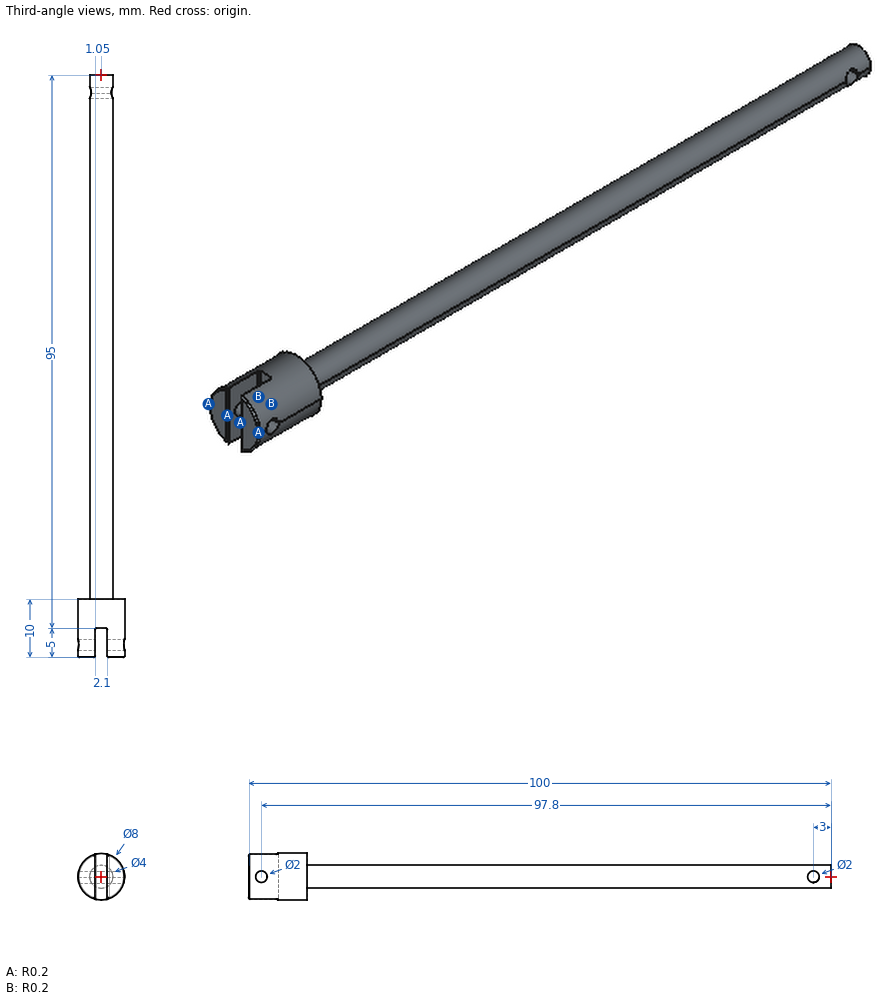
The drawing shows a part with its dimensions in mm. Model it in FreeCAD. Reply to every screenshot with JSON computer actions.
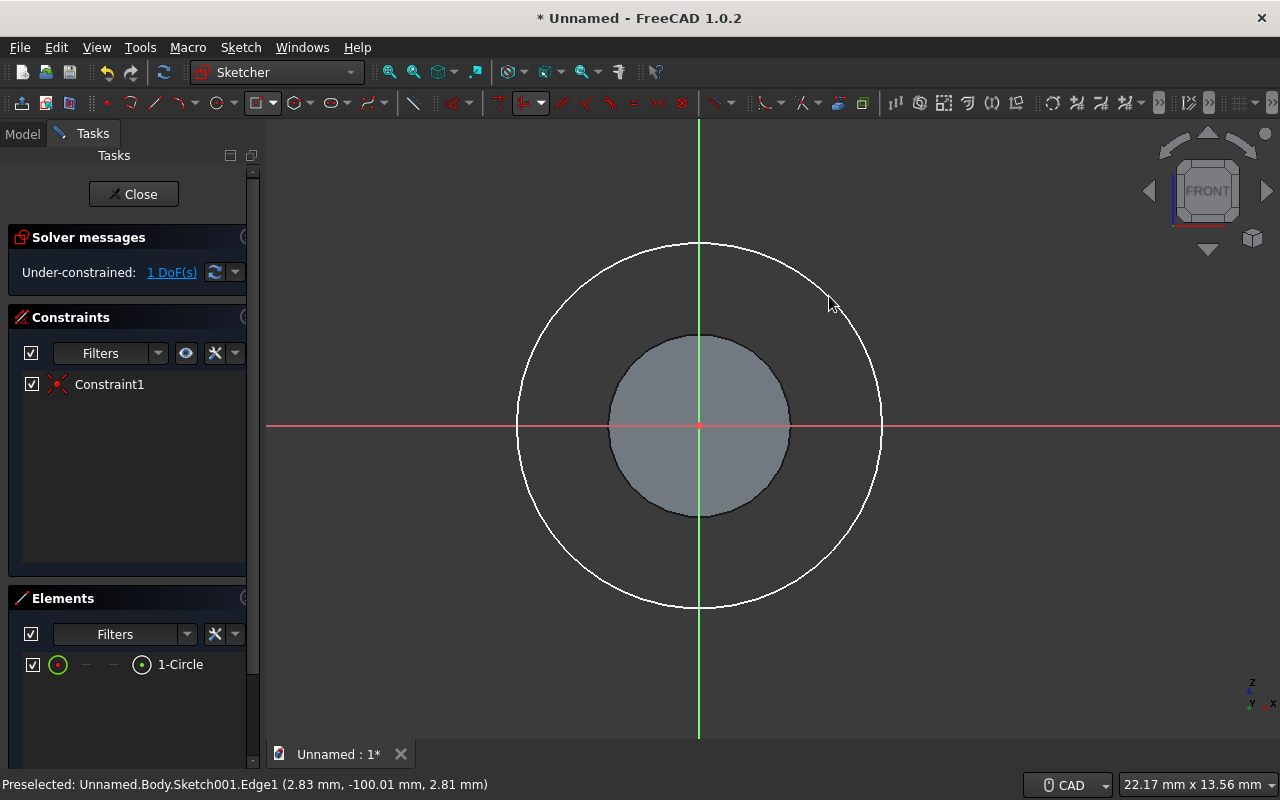
{"action": "key", "text": "d"}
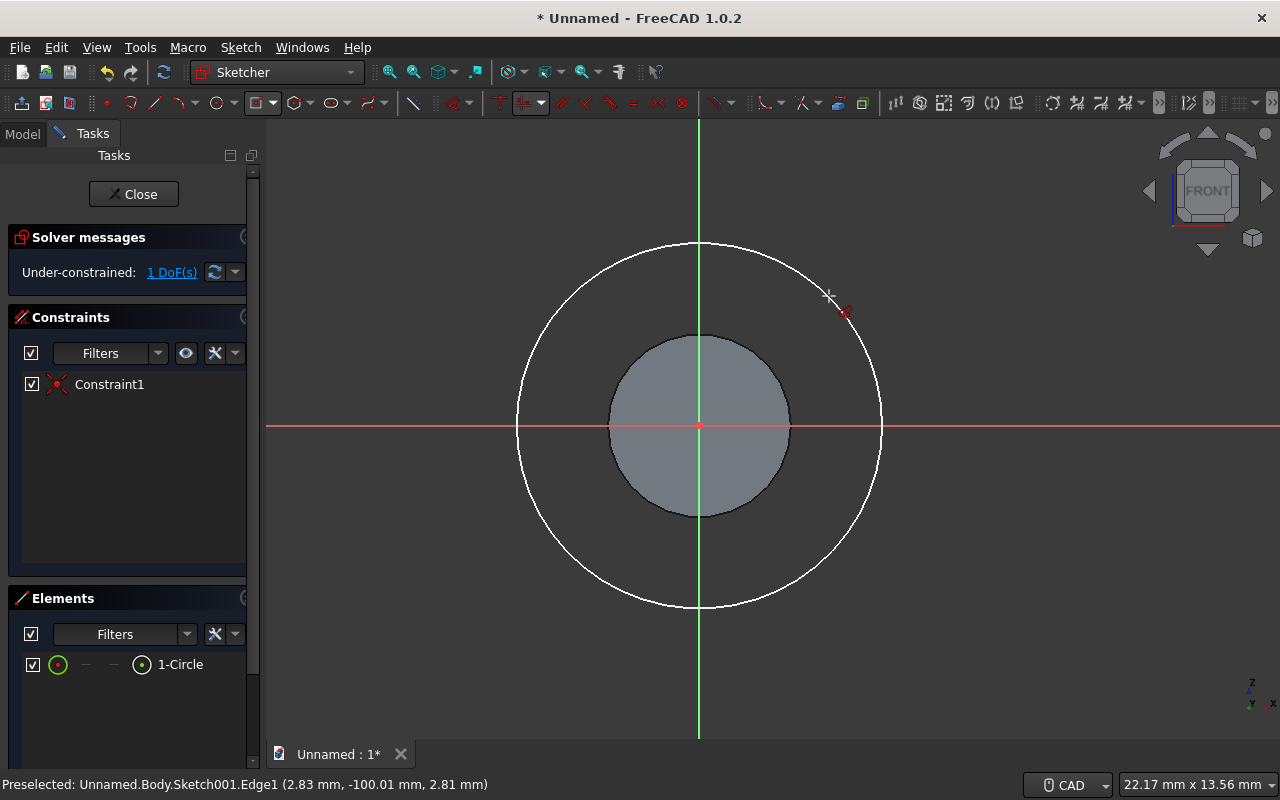
{"action": "left_click", "coordinate": [828, 296]}
{"action": "left_click", "coordinate": [851, 273]}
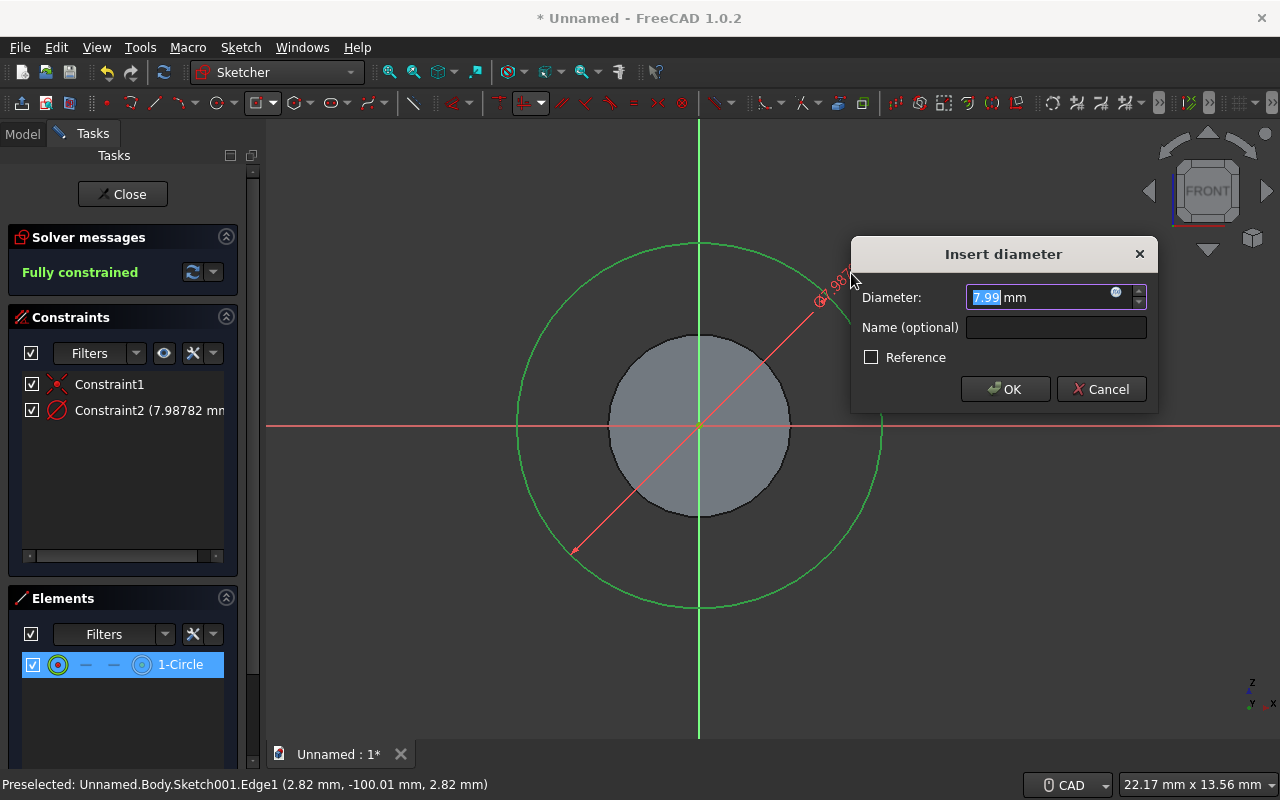
{"action": "type", "text": "8"}
{"action": "key", "text": "Return"}
{"action": "key", "text": "Escape"}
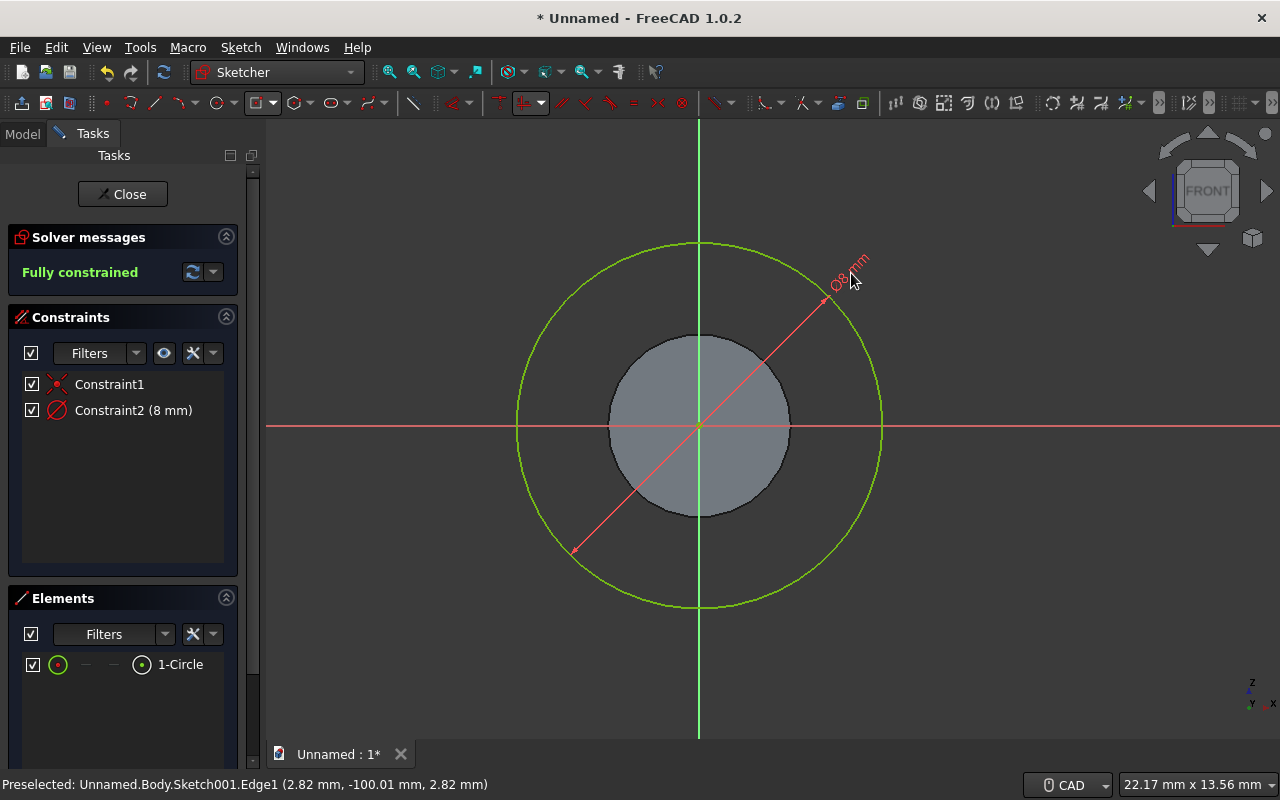
{"action": "left_click", "coordinate": [123, 194]}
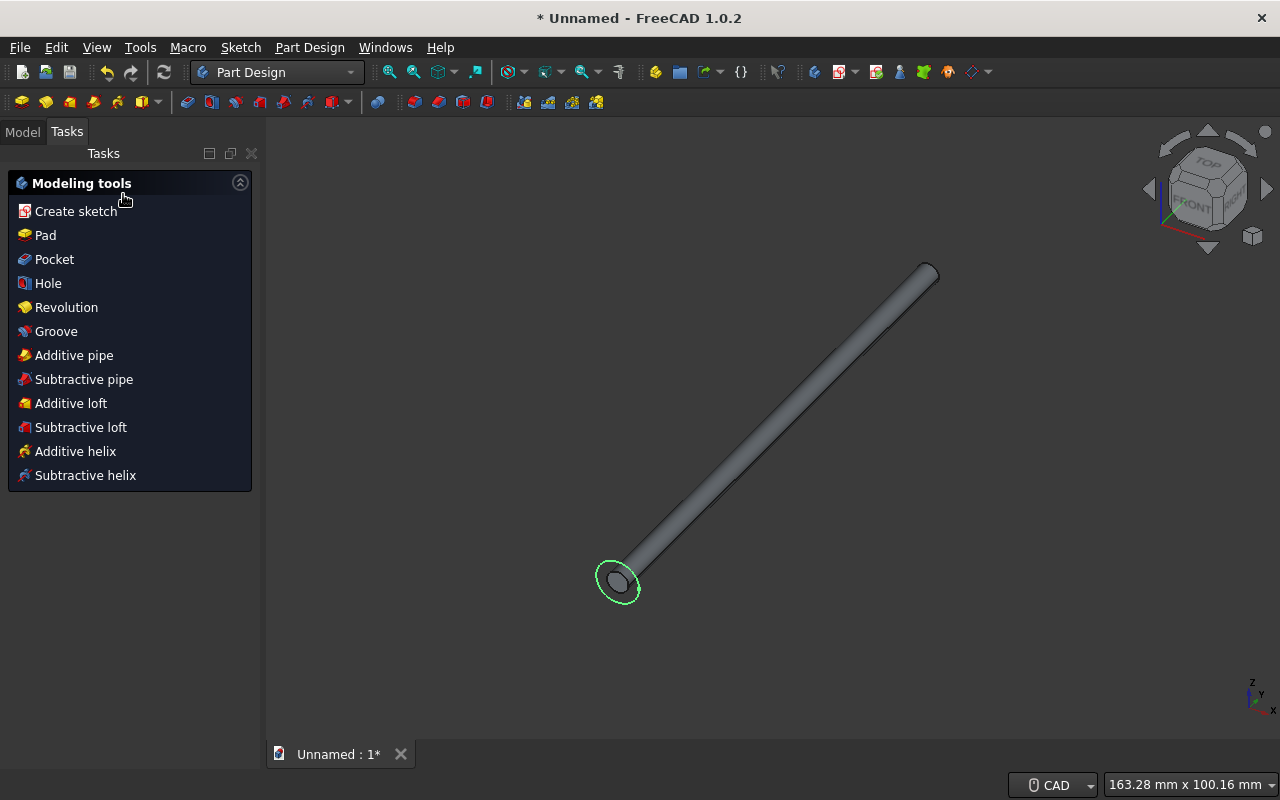
{"action": "left_click", "coordinate": [22, 102]}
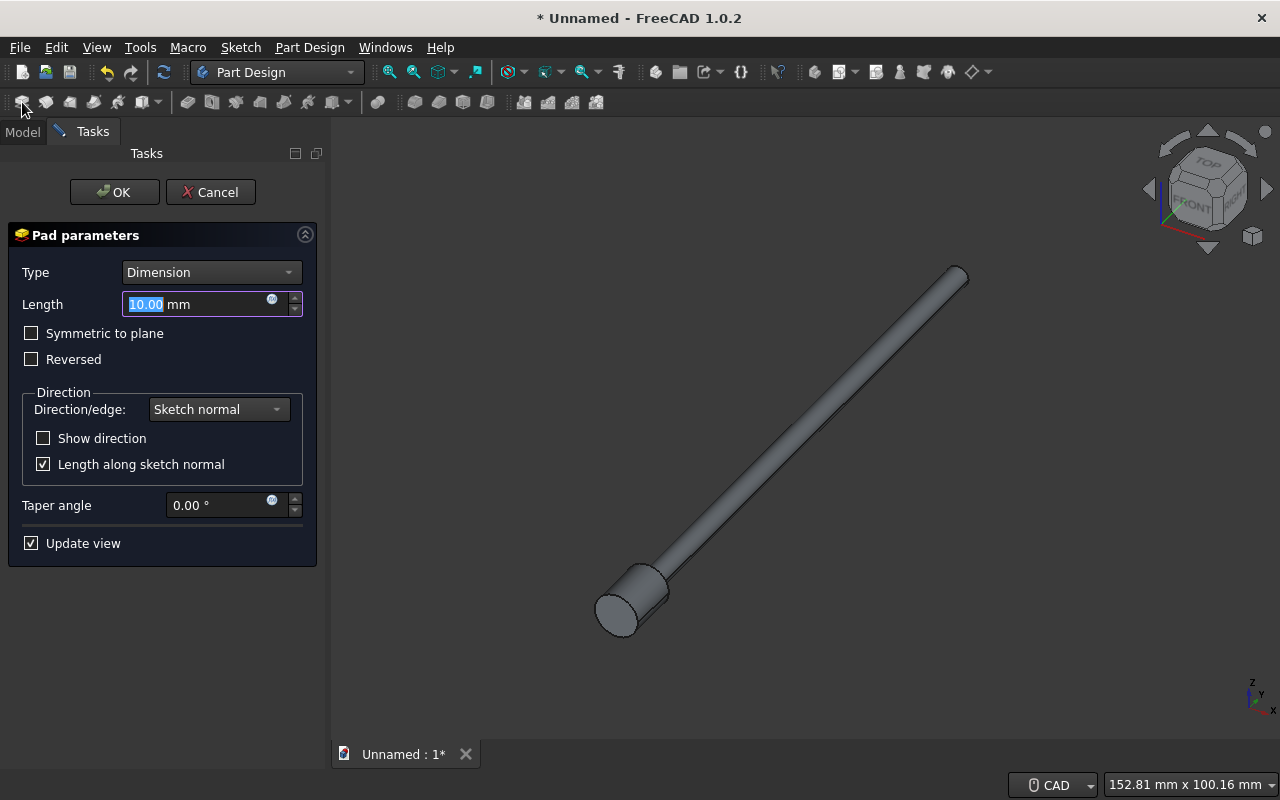
{"action": "type", "text": "10"}
{"action": "key", "text": "Tab"}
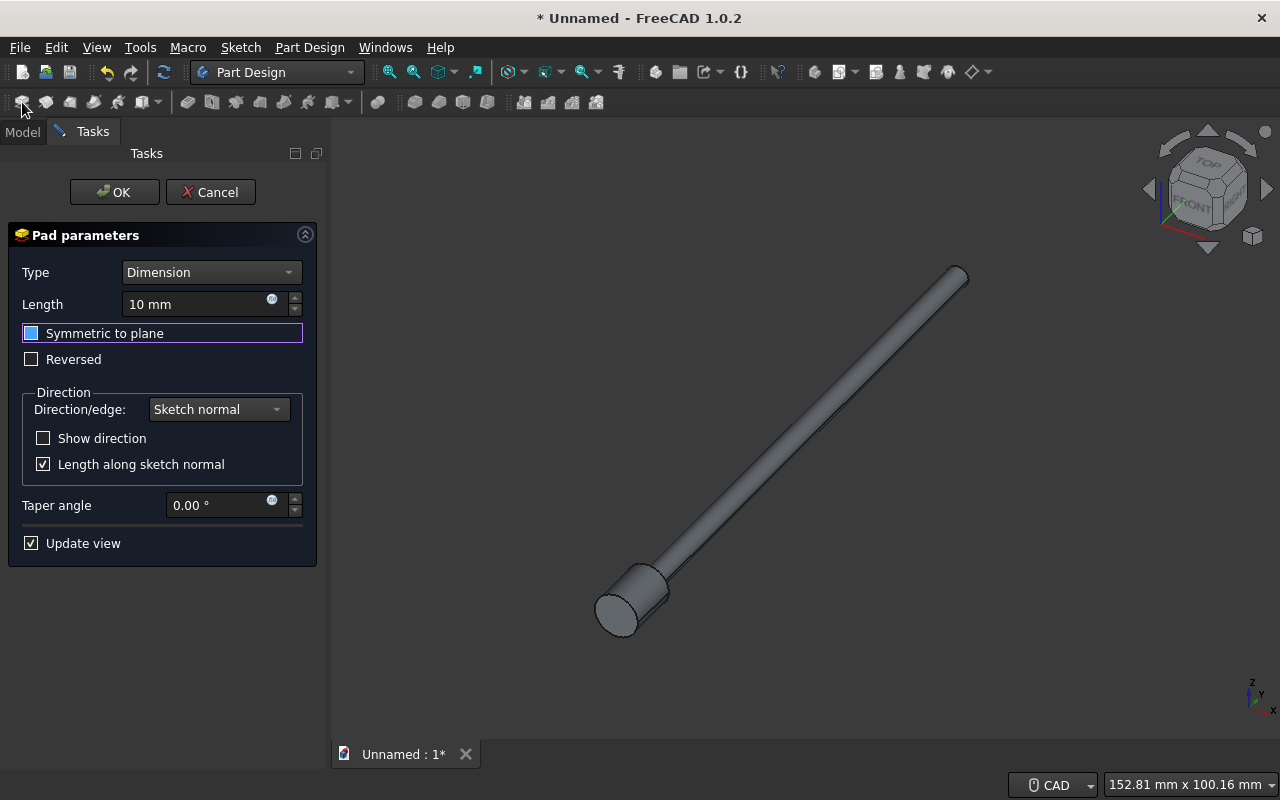
{"action": "left_click", "coordinate": [30, 359]}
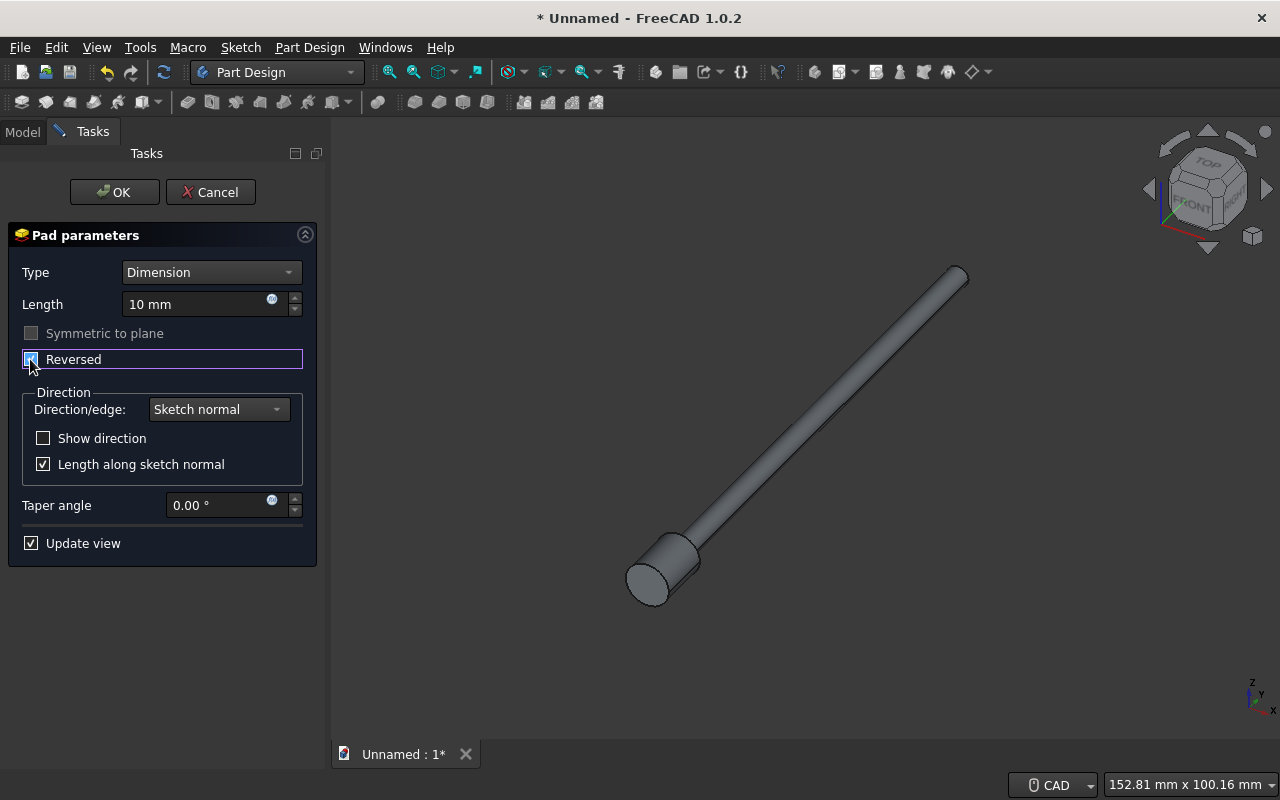
{"action": "left_click", "coordinate": [115, 192]}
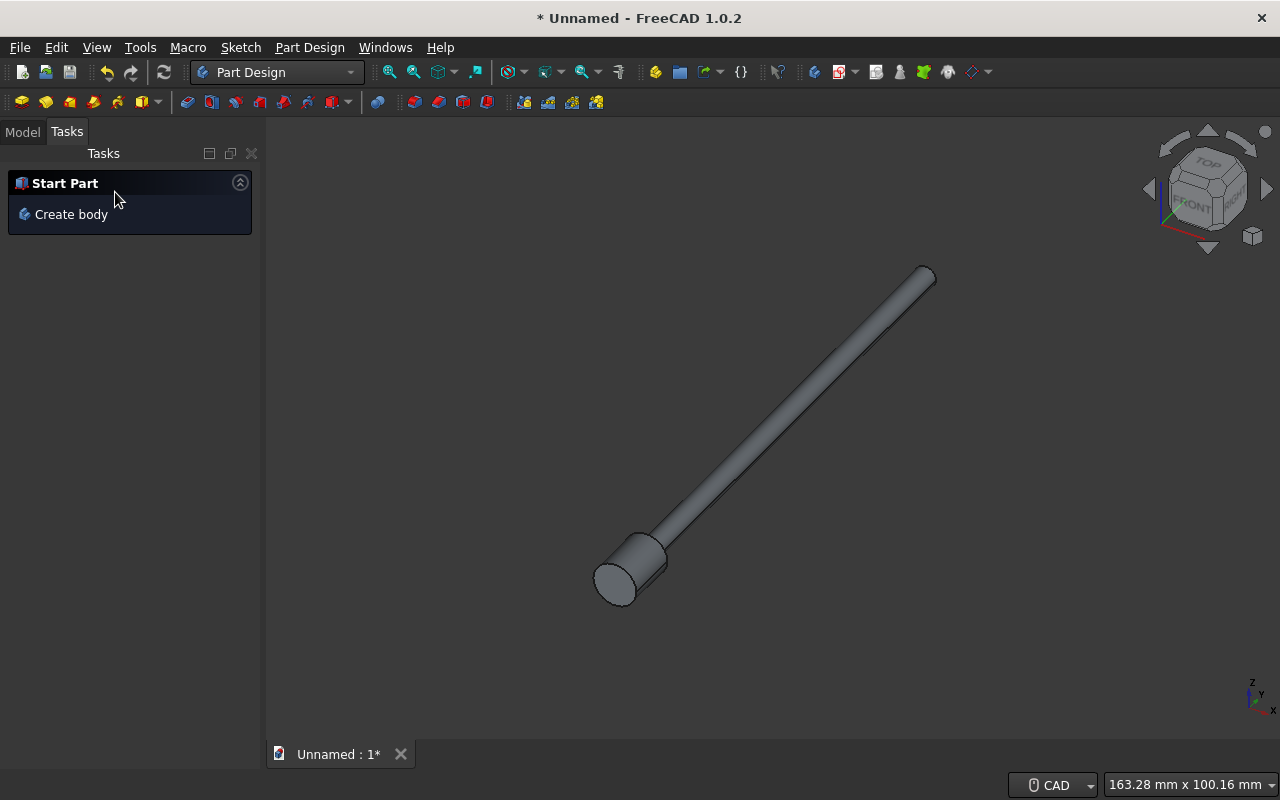
{"action": "left_click", "coordinate": [840, 72]}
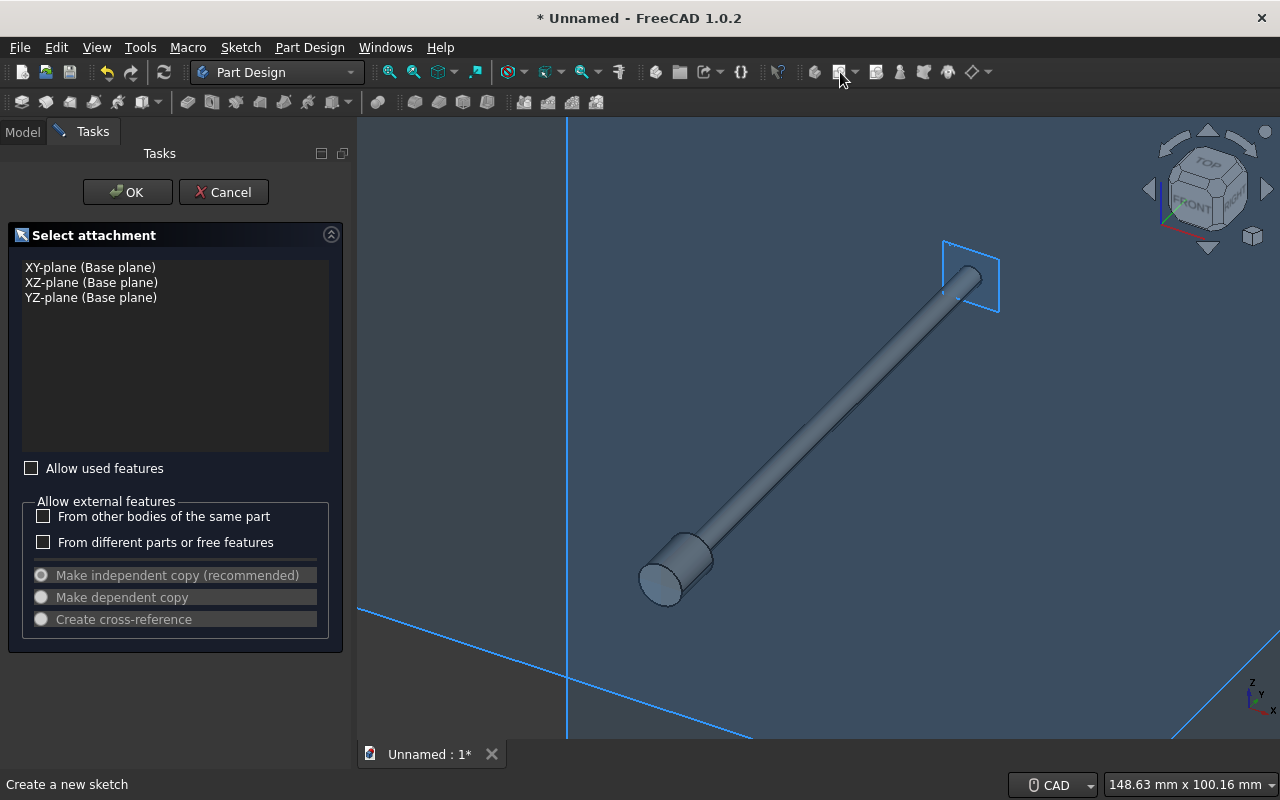
{"action": "left_click", "coordinate": [82, 268]}